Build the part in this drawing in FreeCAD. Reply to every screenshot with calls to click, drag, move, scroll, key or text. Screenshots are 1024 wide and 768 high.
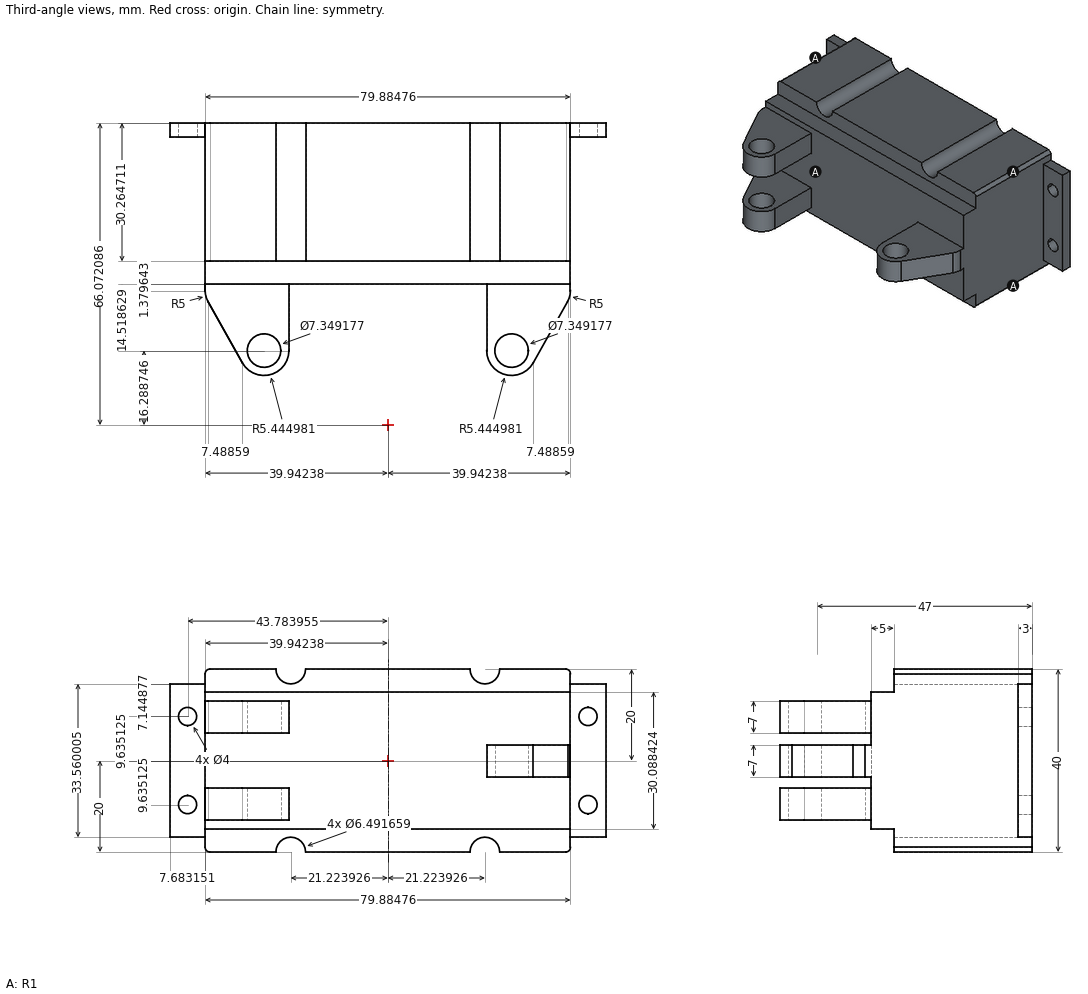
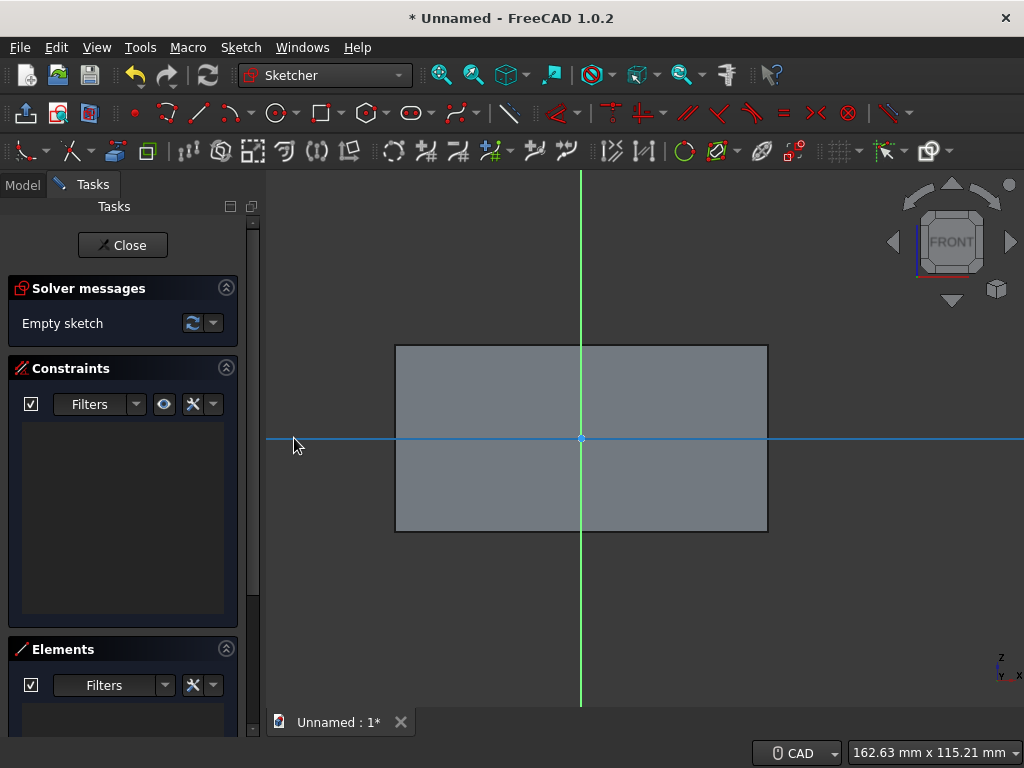
key(g)
key(v)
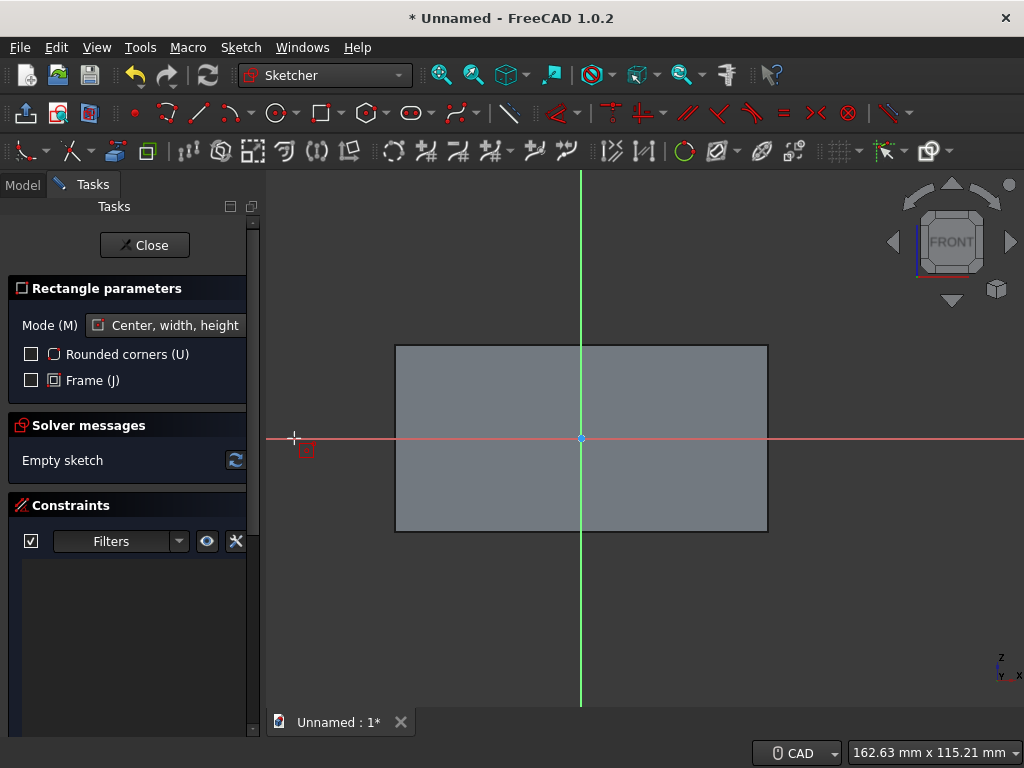
click(581, 439)
click(768, 368)
key(Escape)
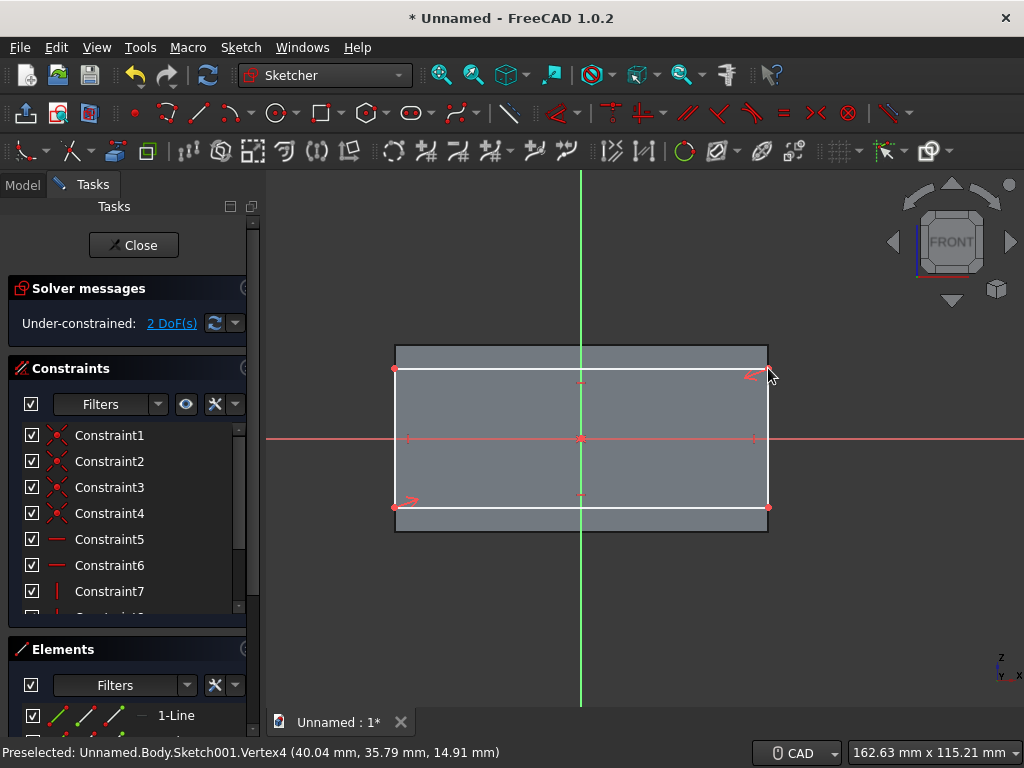
click(556, 114)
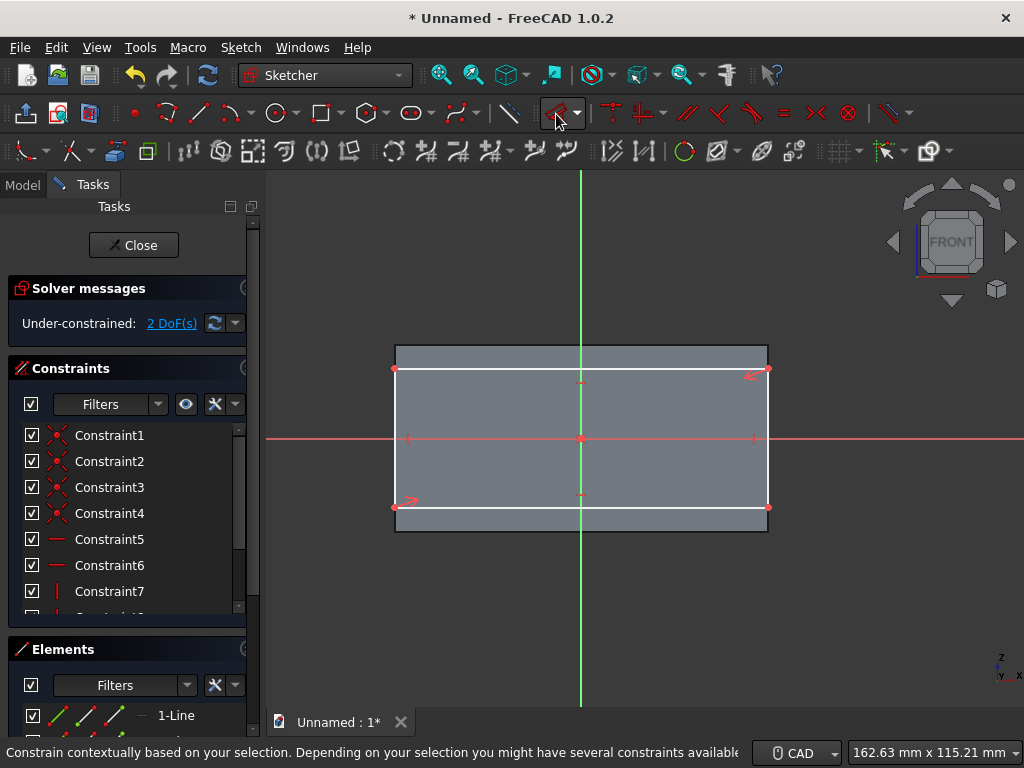
click(507, 508)
click(496, 542)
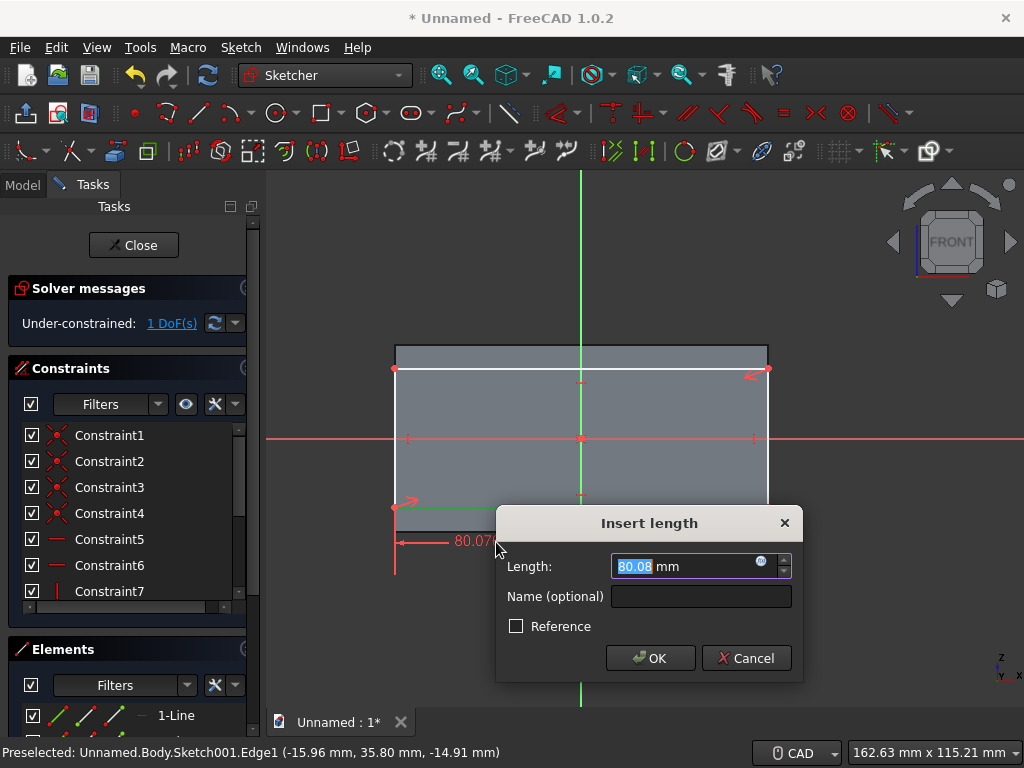
text(79.88476)
key(Return)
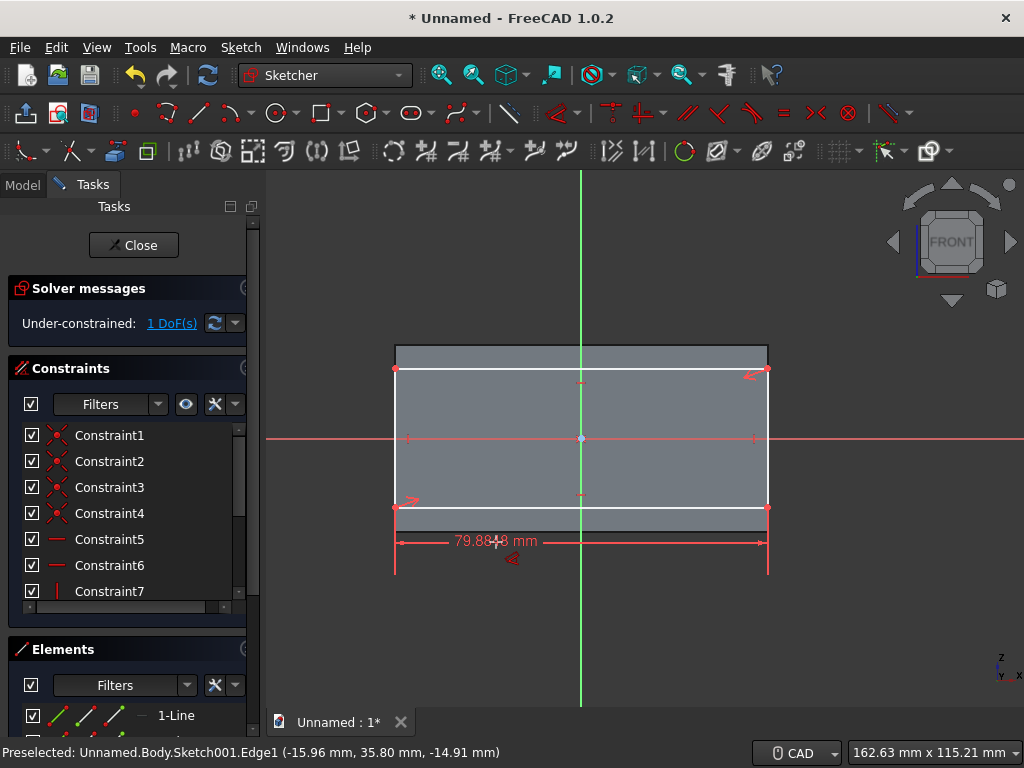
click(768, 466)
click(802, 407)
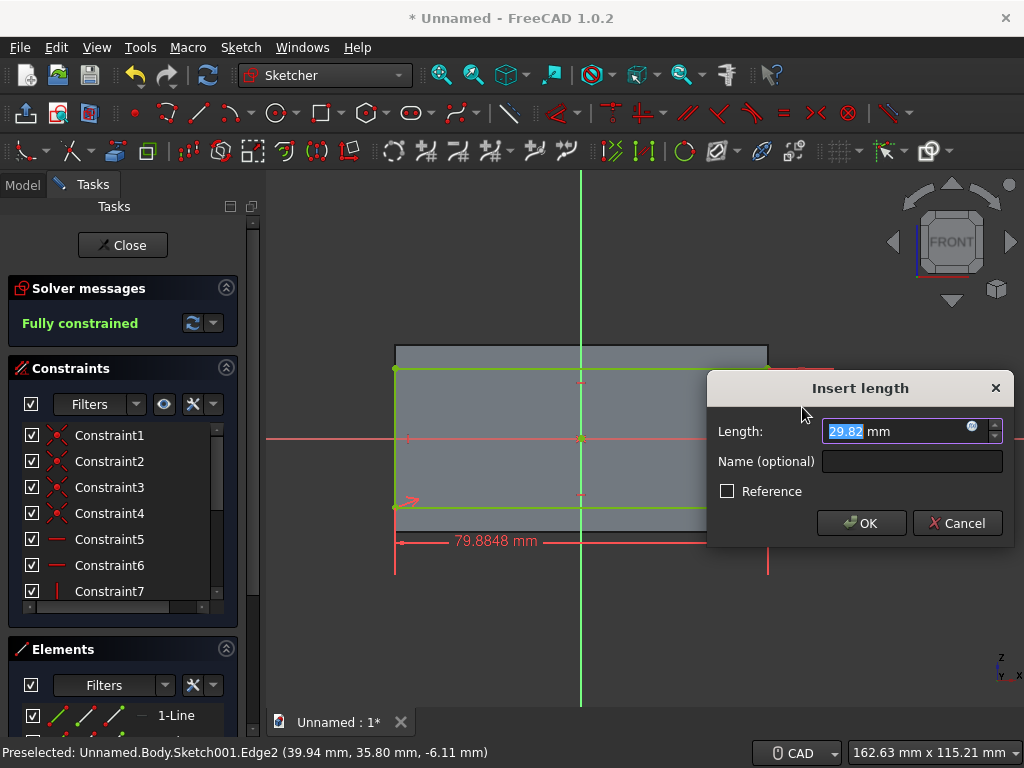
text(30.088424)
key(Return)
key(Escape)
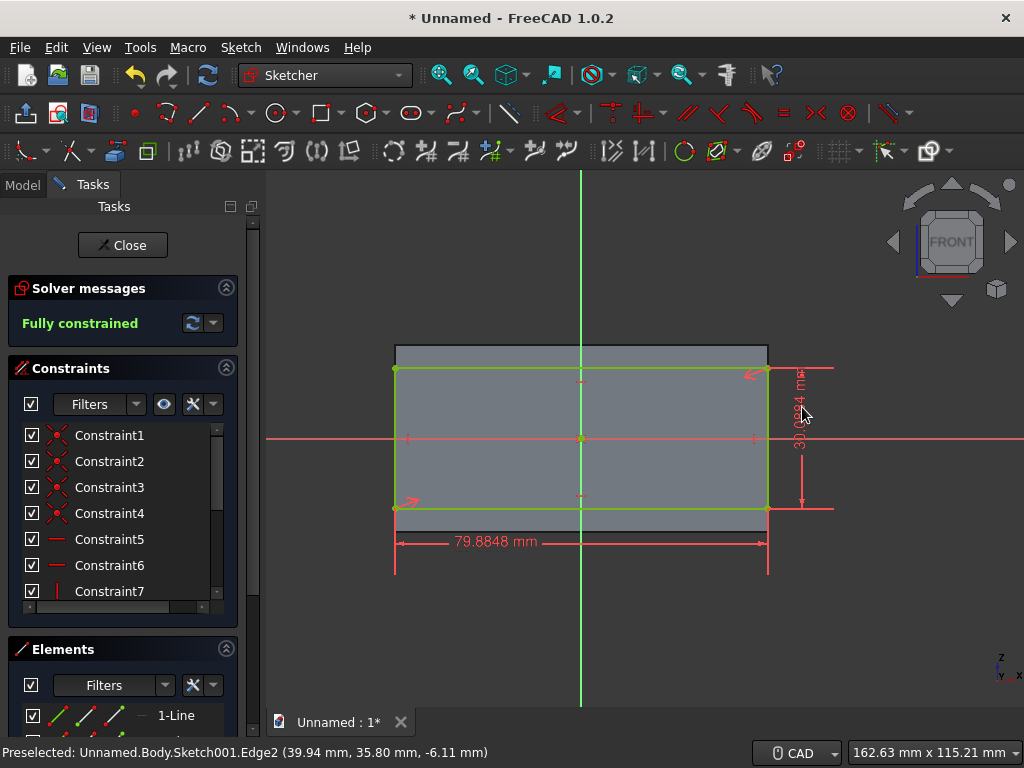
click(123, 245)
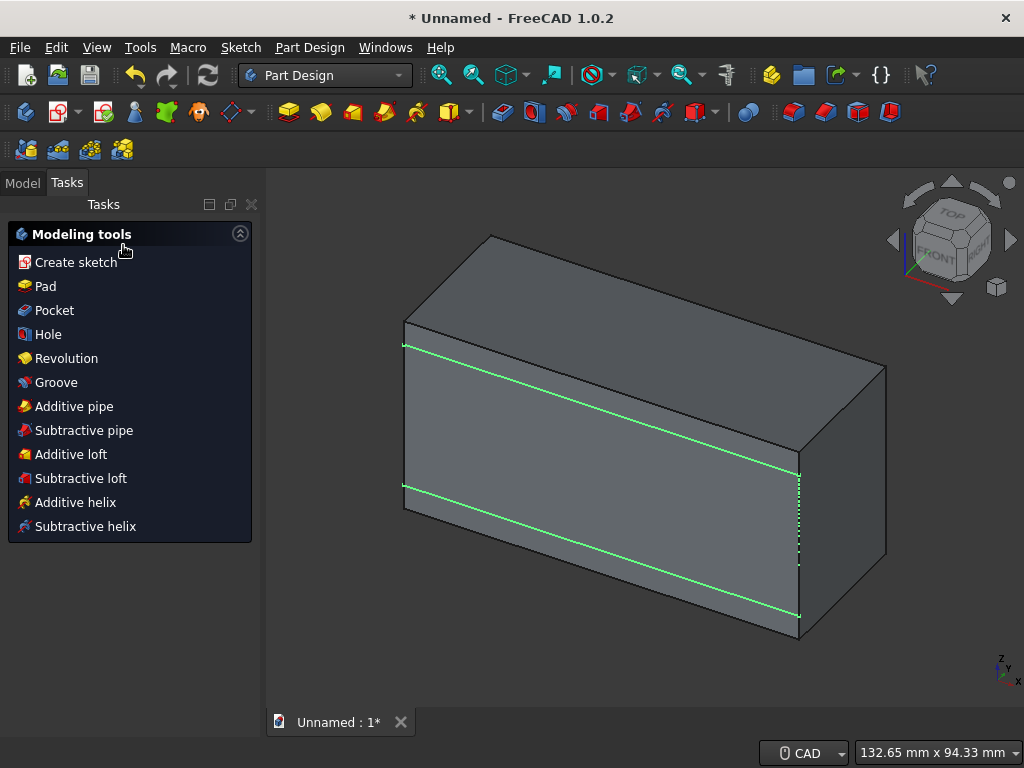
click(290, 112)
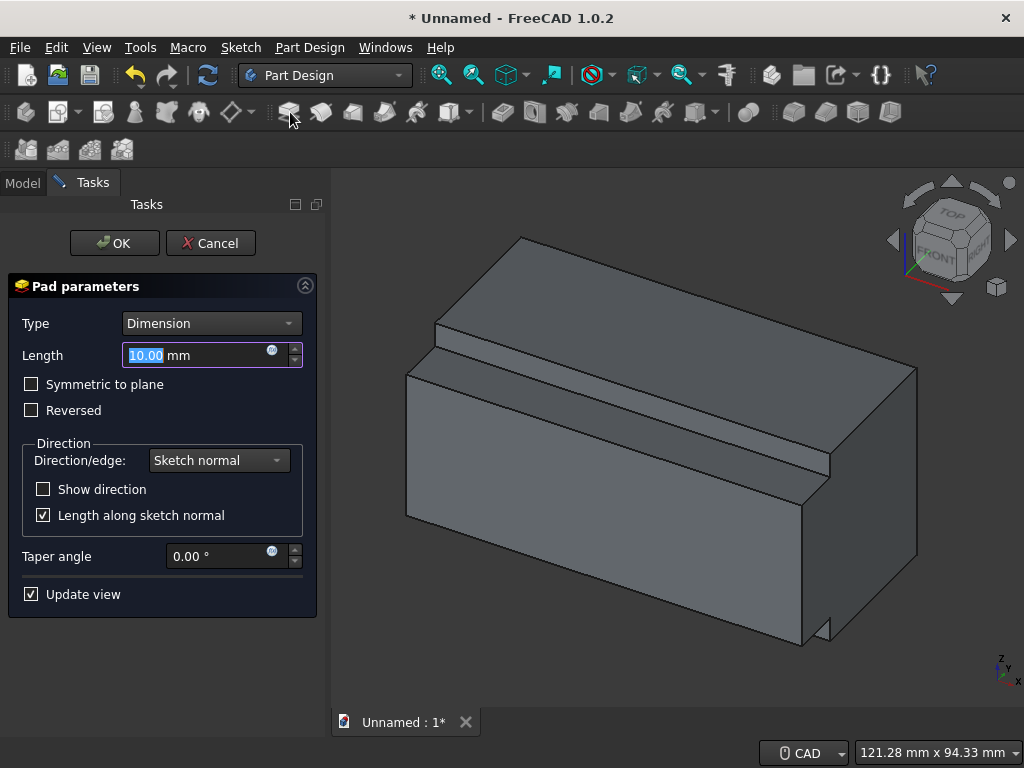
text(5)
key(Tab)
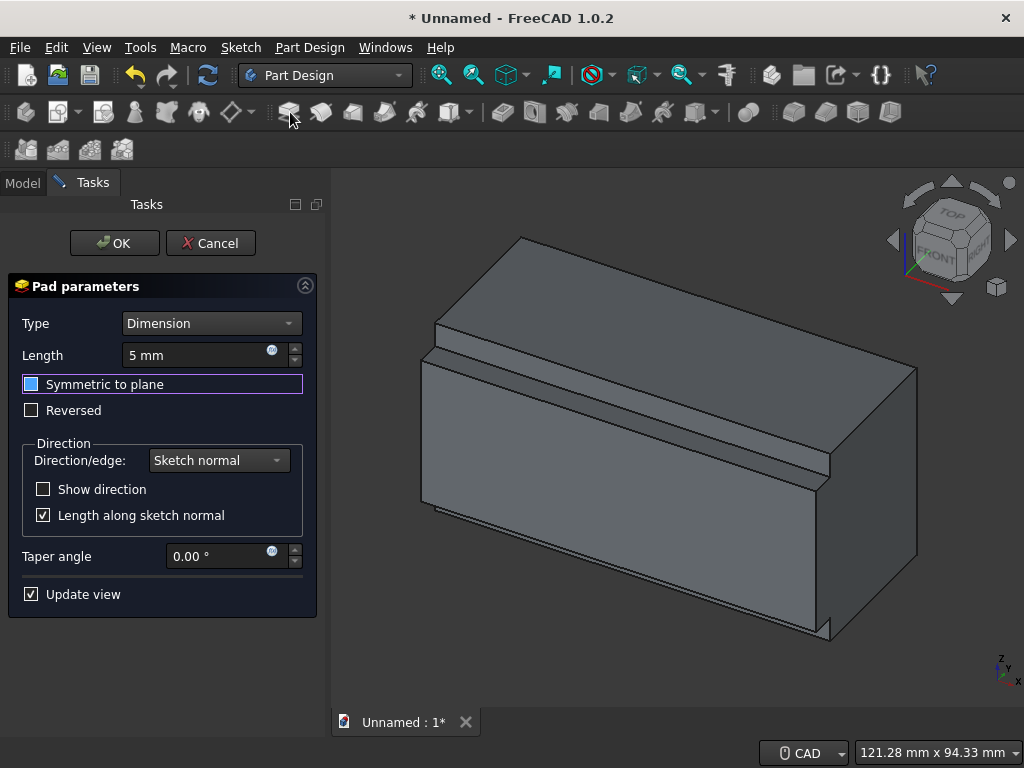
click(115, 243)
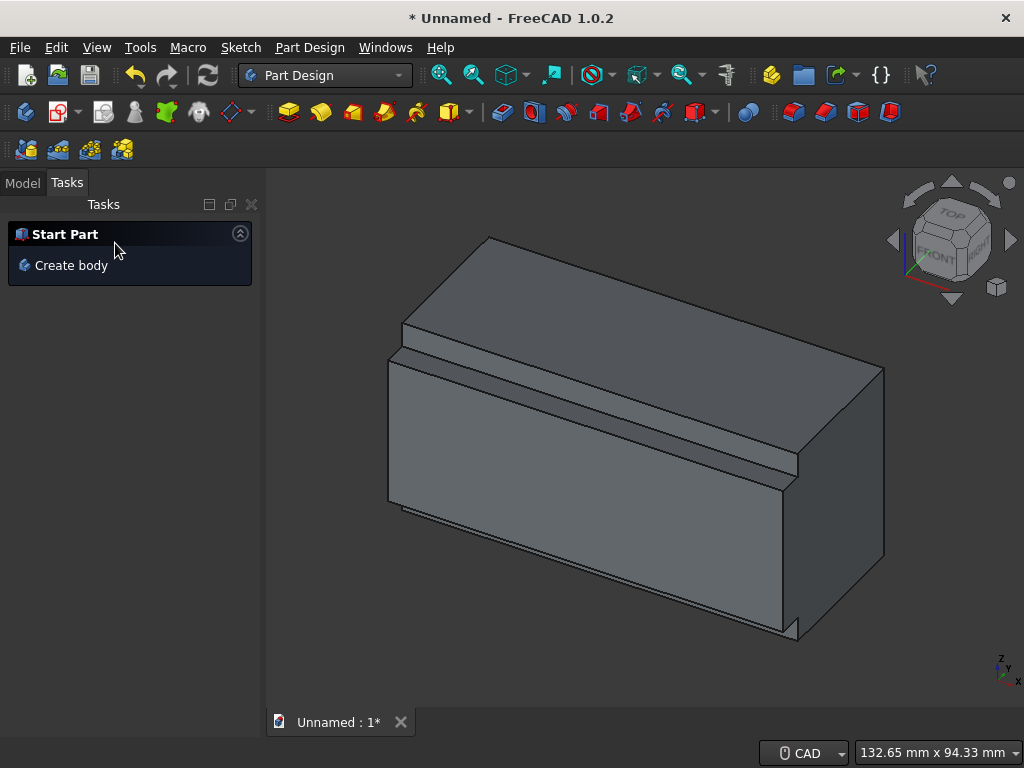
key(4)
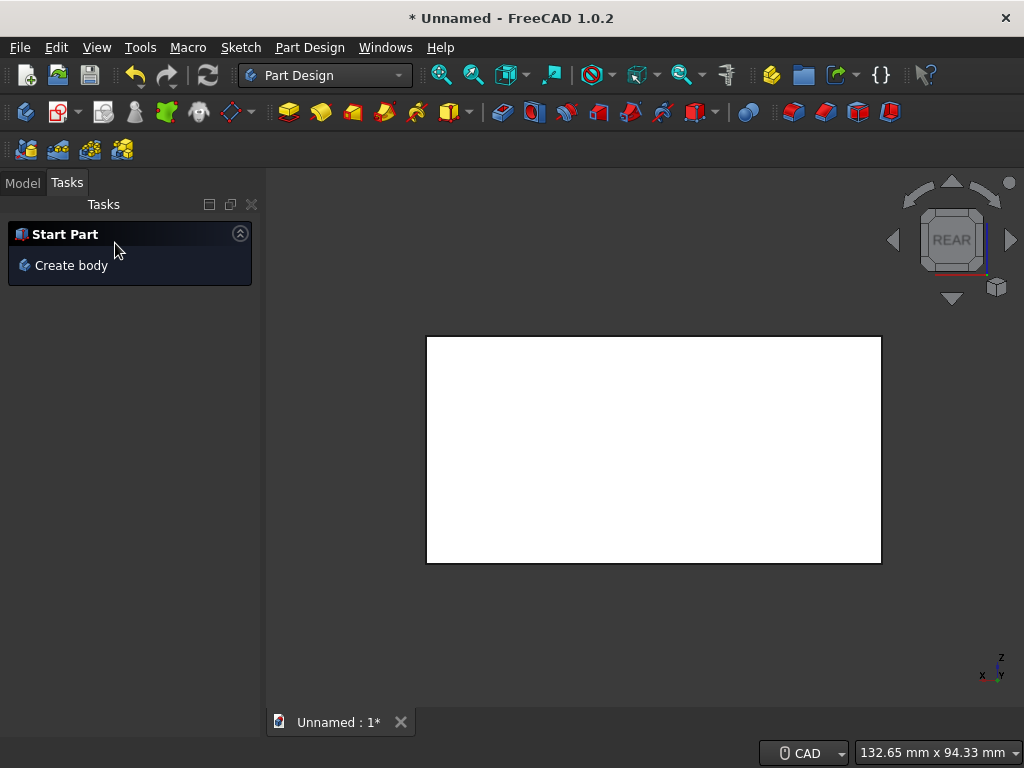
click(589, 449)